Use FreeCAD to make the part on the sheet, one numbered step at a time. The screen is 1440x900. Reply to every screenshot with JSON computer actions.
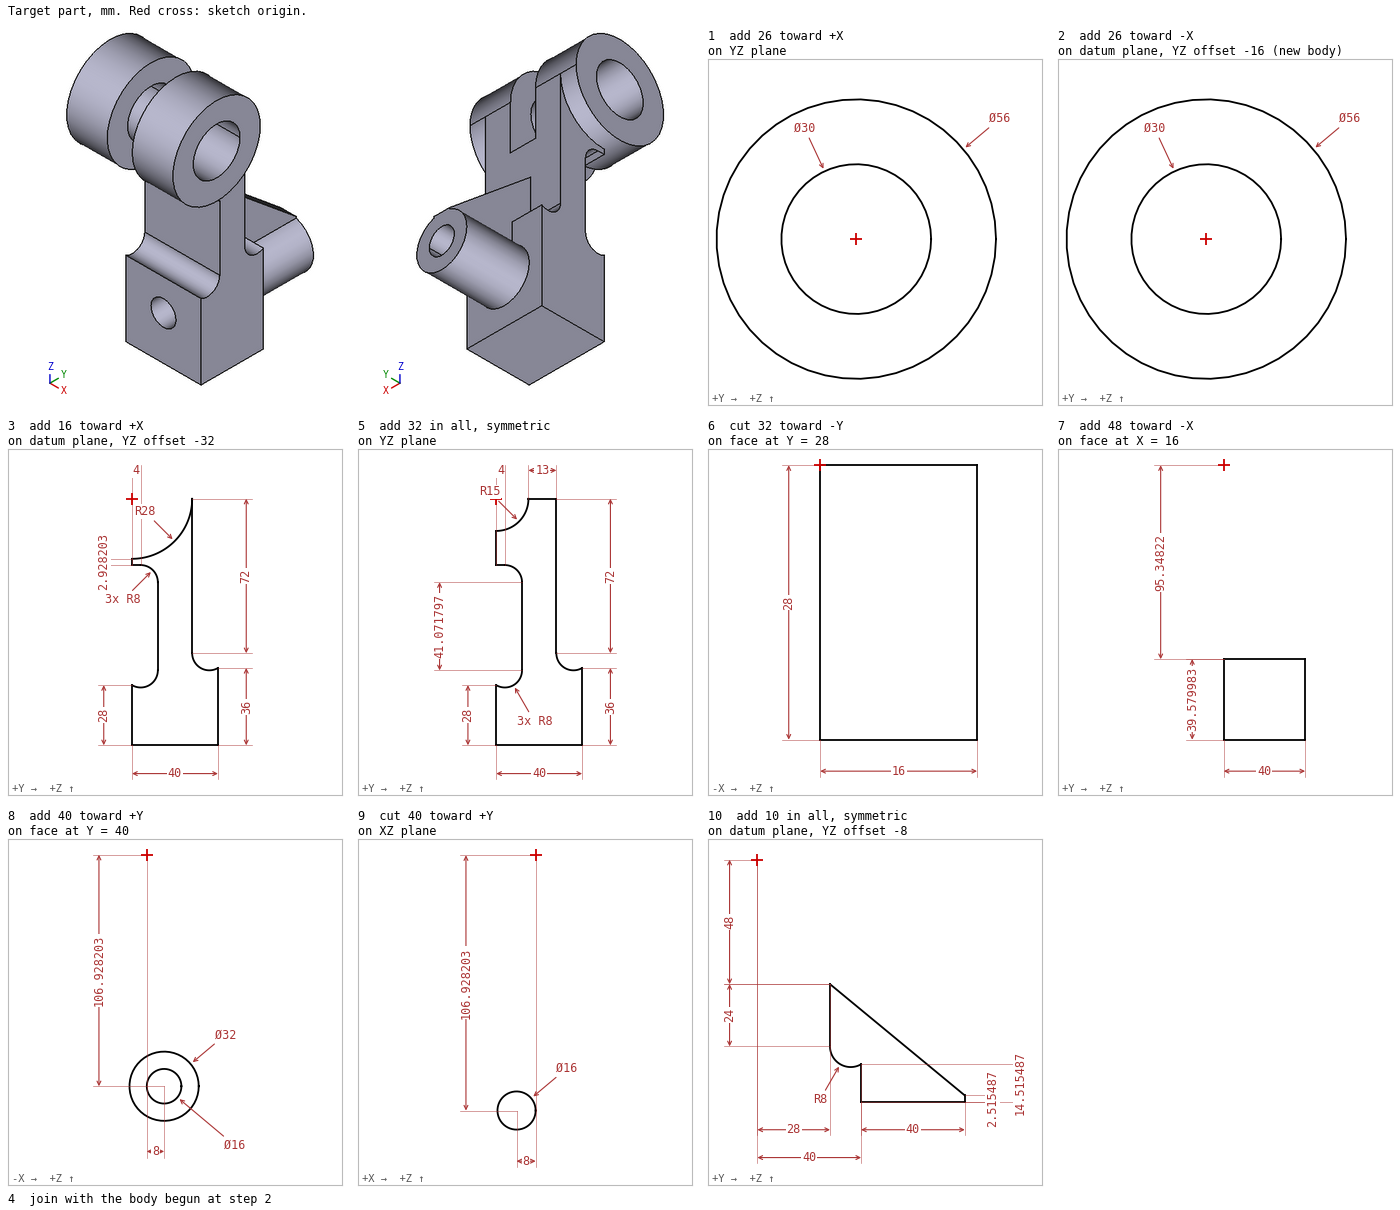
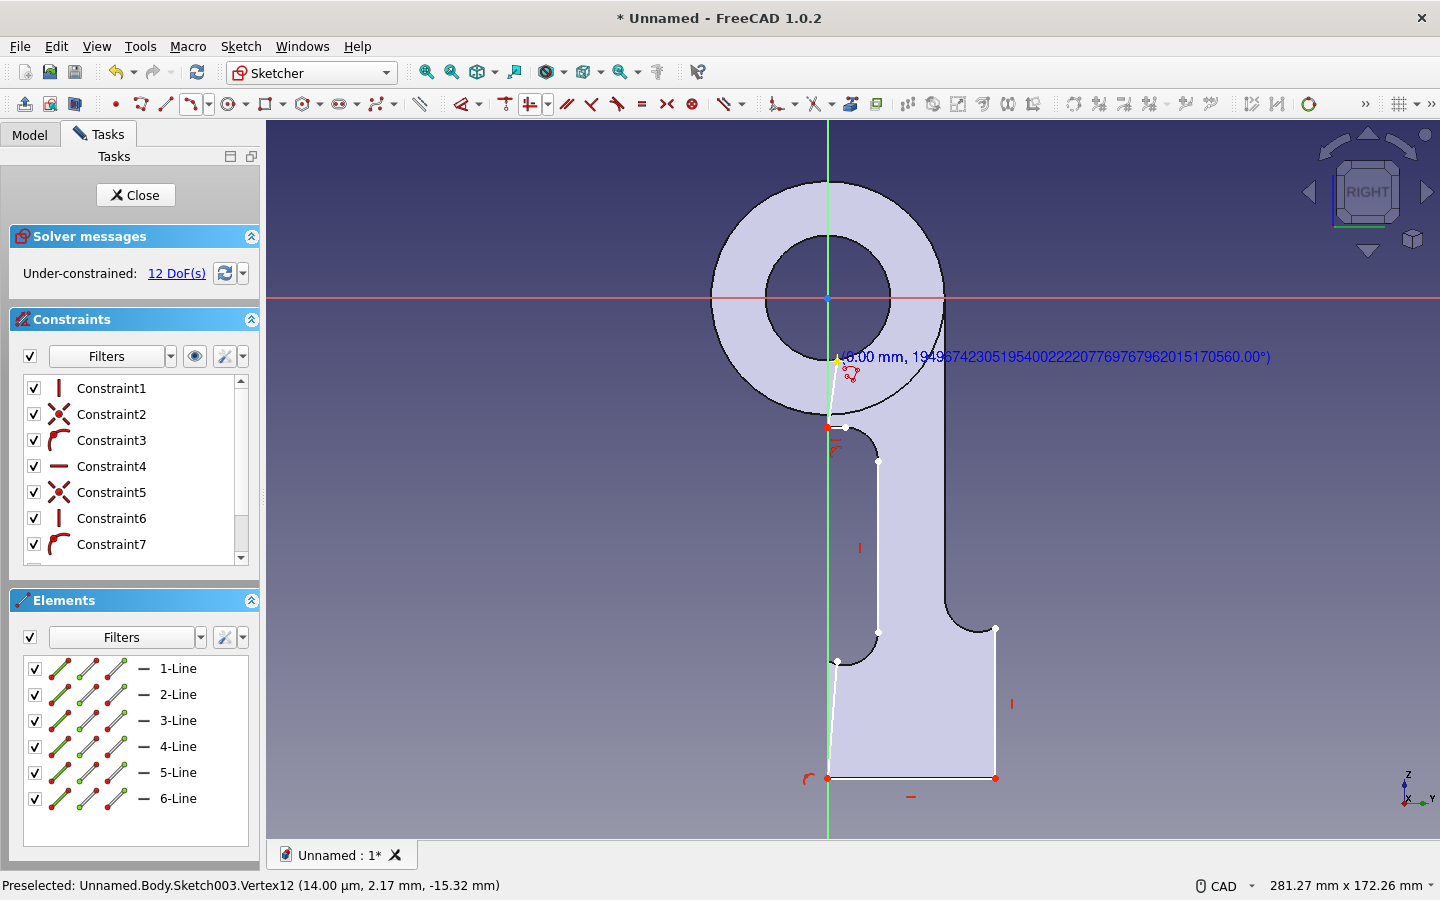
{"action": "left_click", "coordinate": [891, 298]}
{"action": "left_click", "coordinate": [945, 307]}
{"action": "left_click", "coordinate": [945, 599]}
{"action": "right_click", "coordinate": [945, 599]}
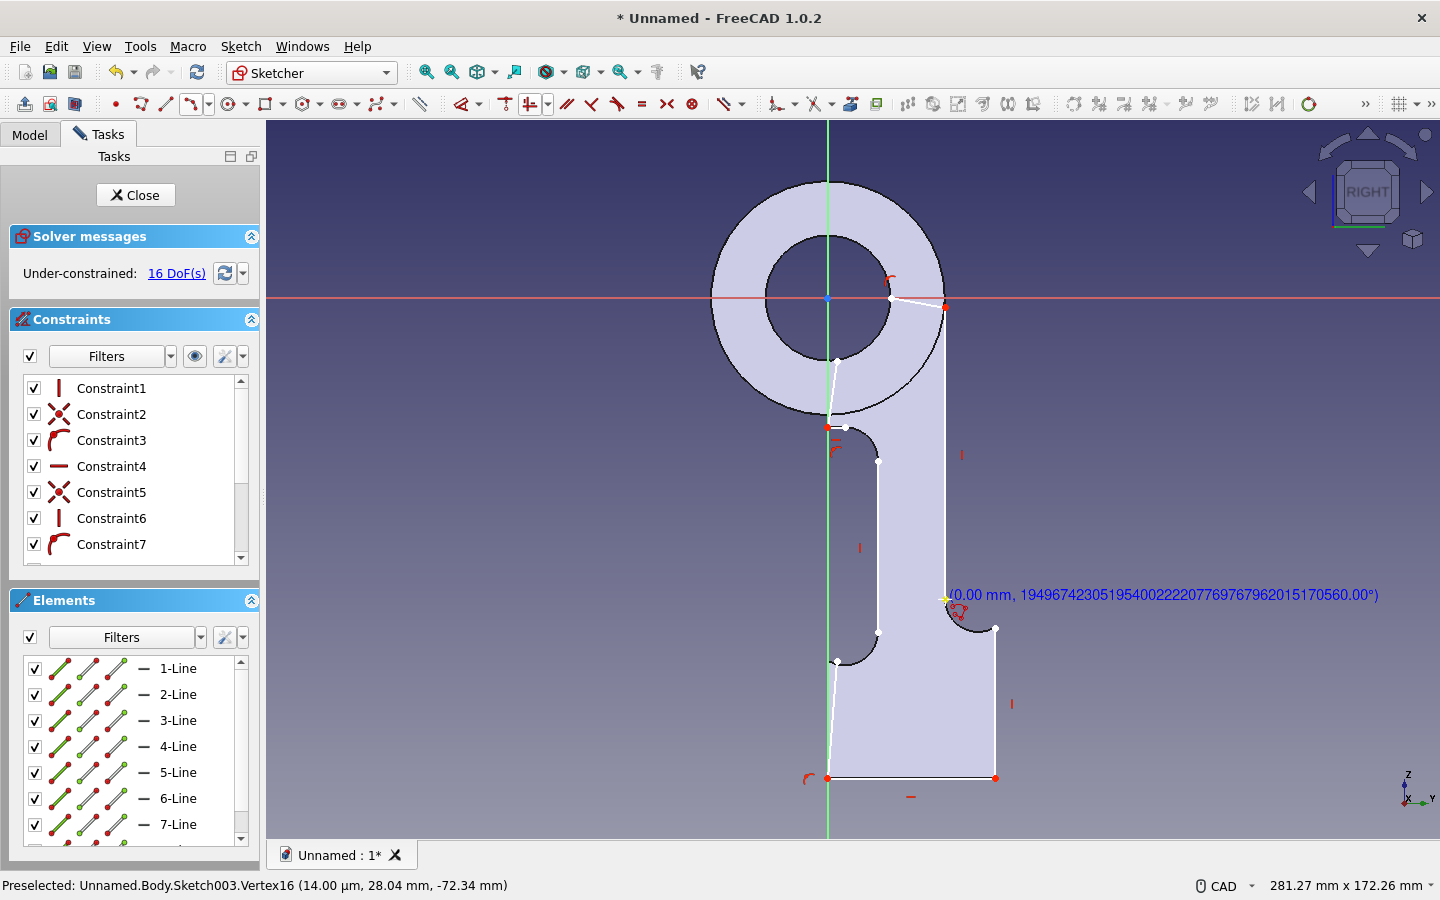
{"action": "left_click", "coordinate": [190, 104]}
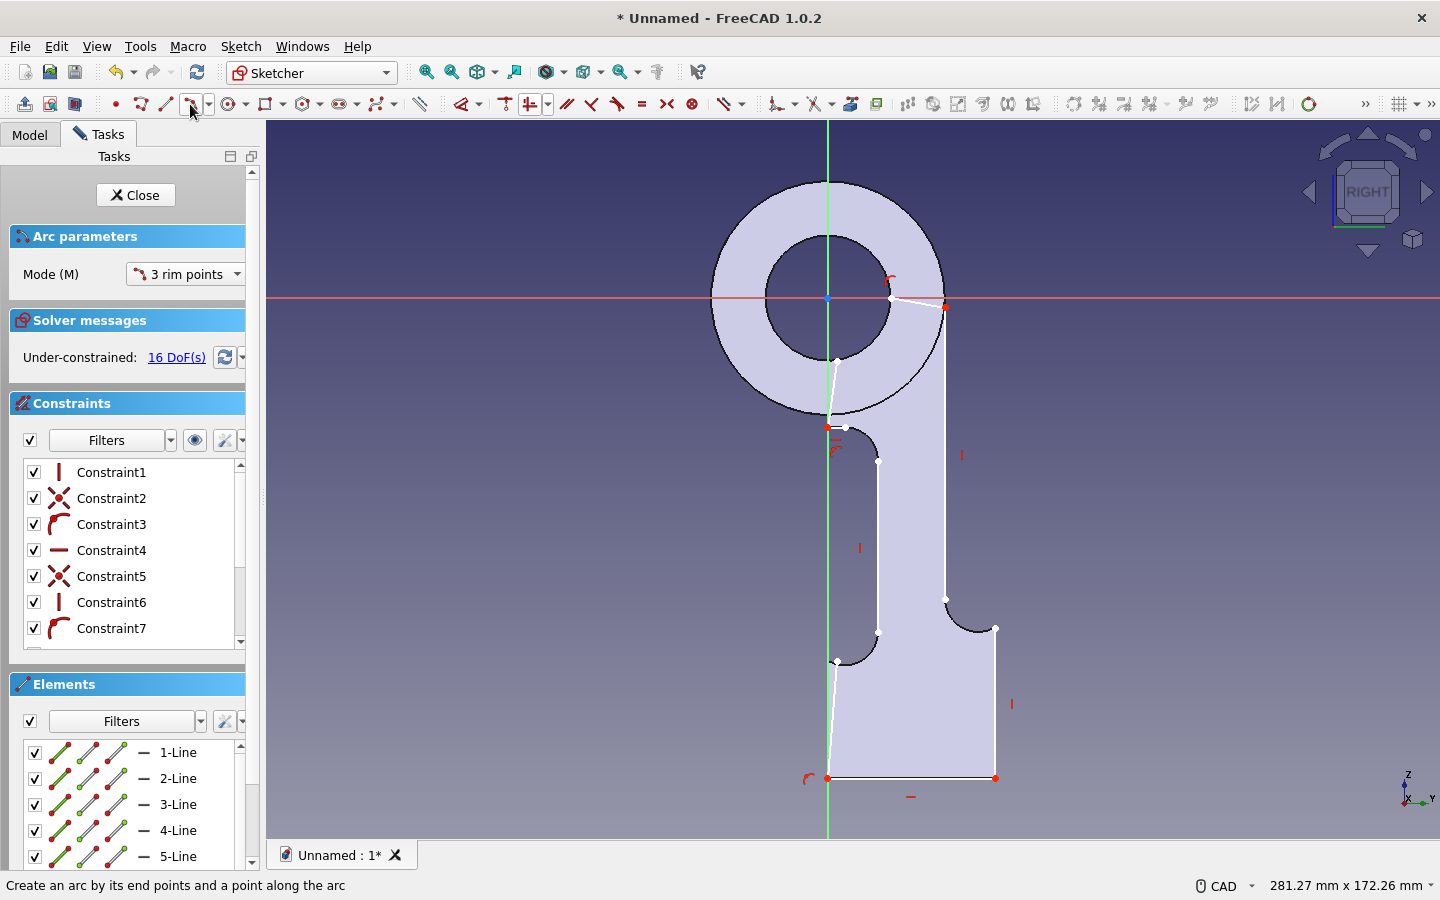
{"action": "left_click", "coordinate": [837, 662]}
{"action": "left_click", "coordinate": [878, 633]}
{"action": "left_click", "coordinate": [861, 661]}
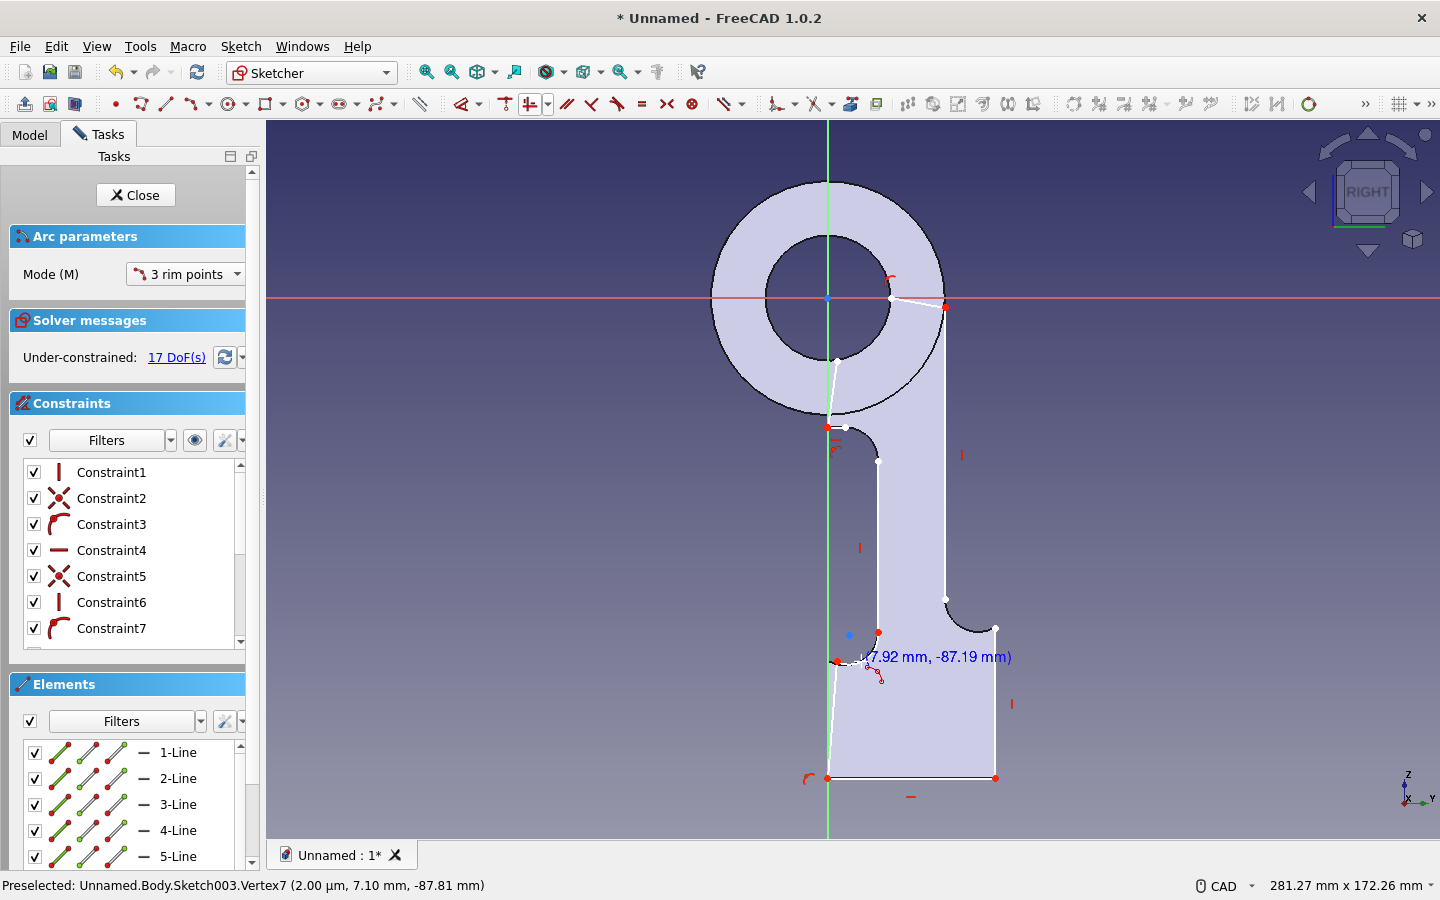
{"action": "left_click", "coordinate": [878, 462]}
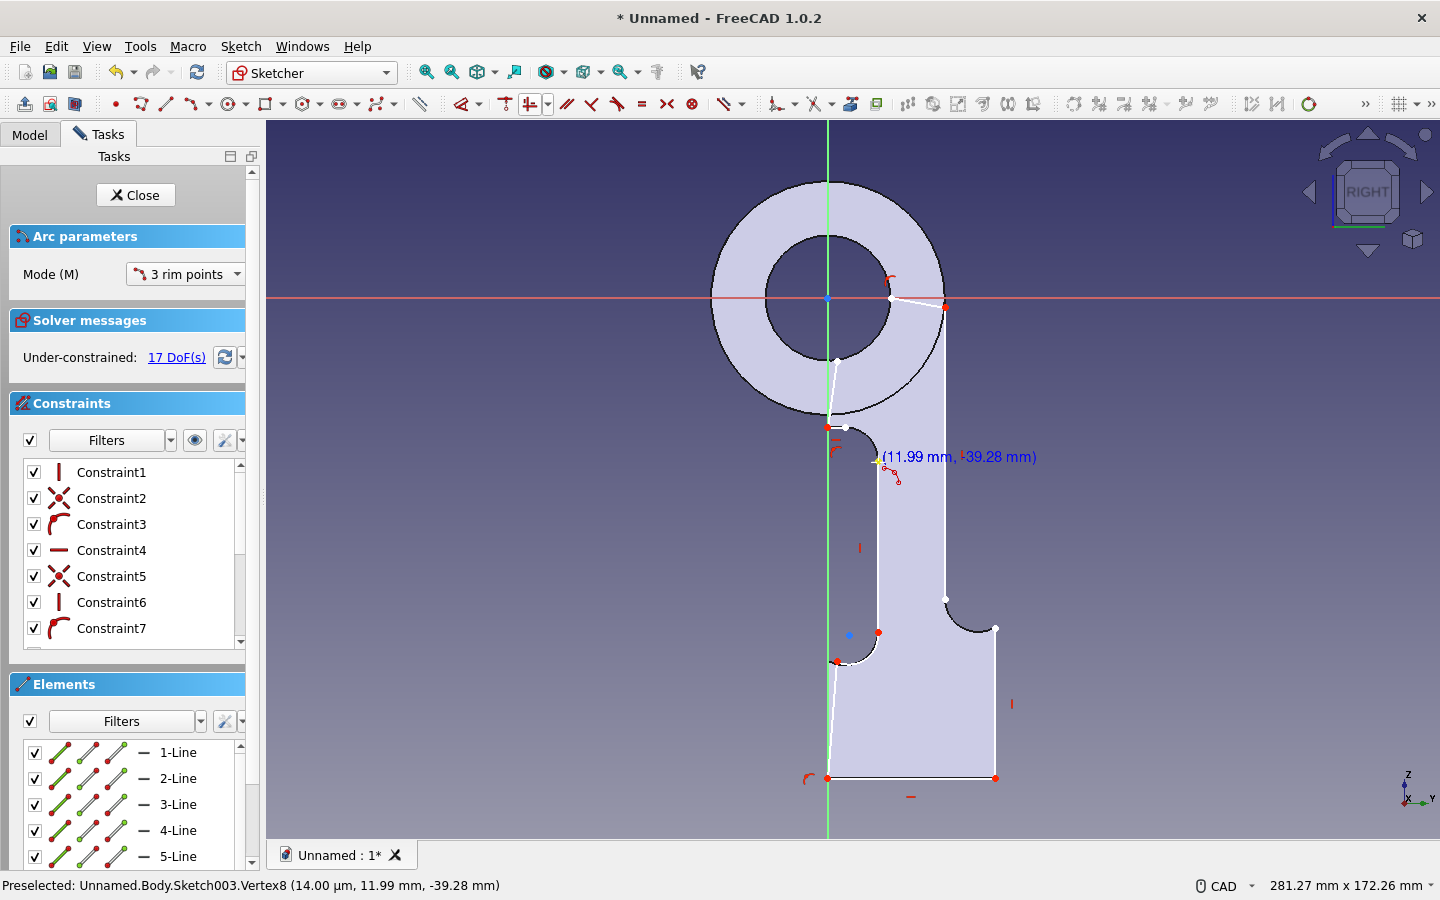
{"action": "scroll", "coordinate": [845, 427], "scroll_direction": "up", "scroll_amount": 4}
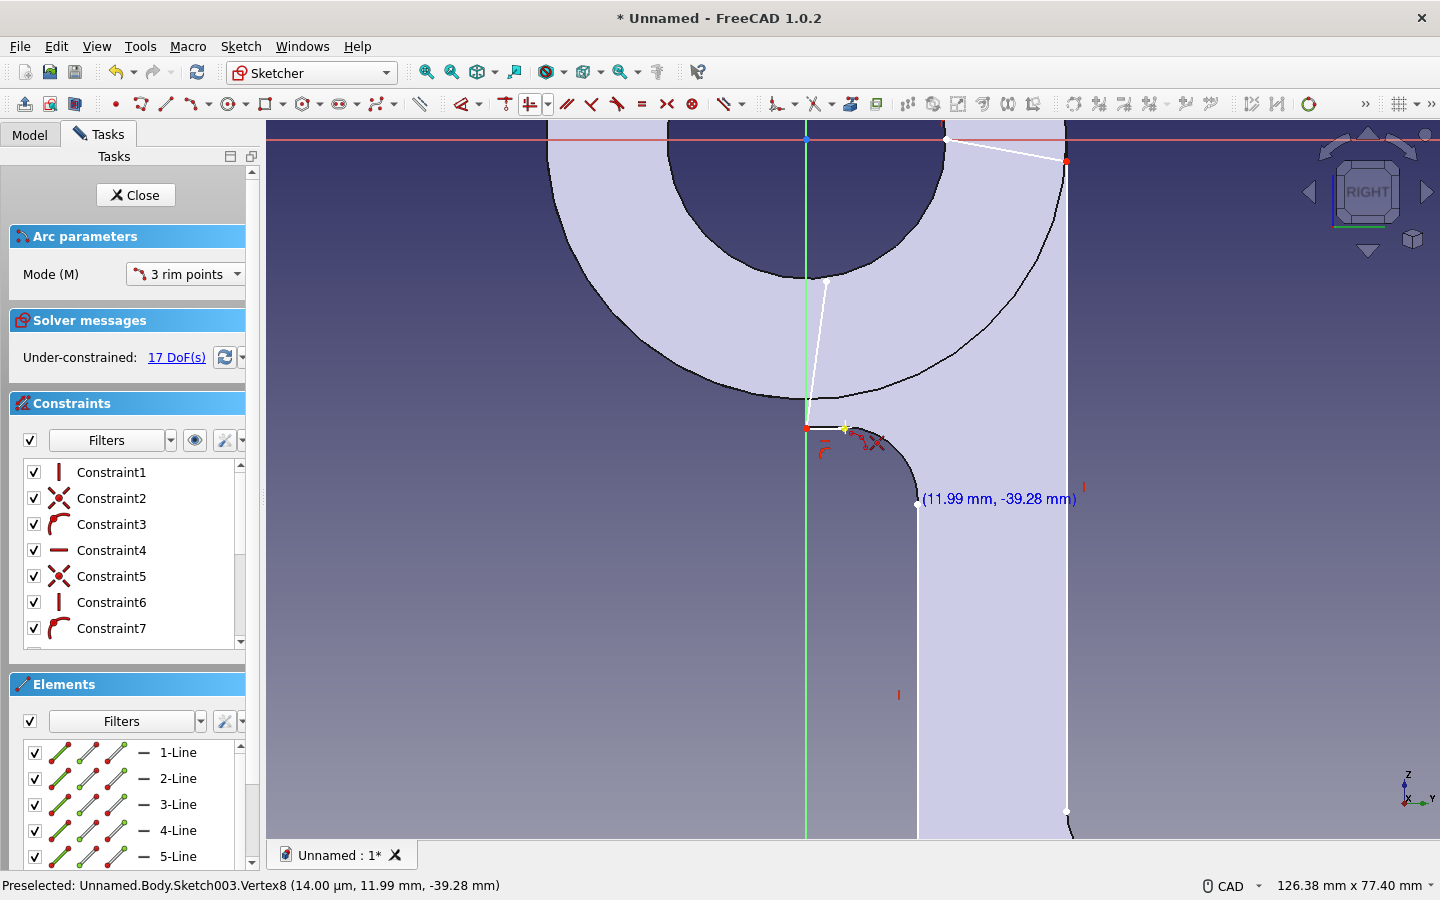
{"action": "left_click", "coordinate": [844, 429]}
{"action": "left_click", "coordinate": [896, 449]}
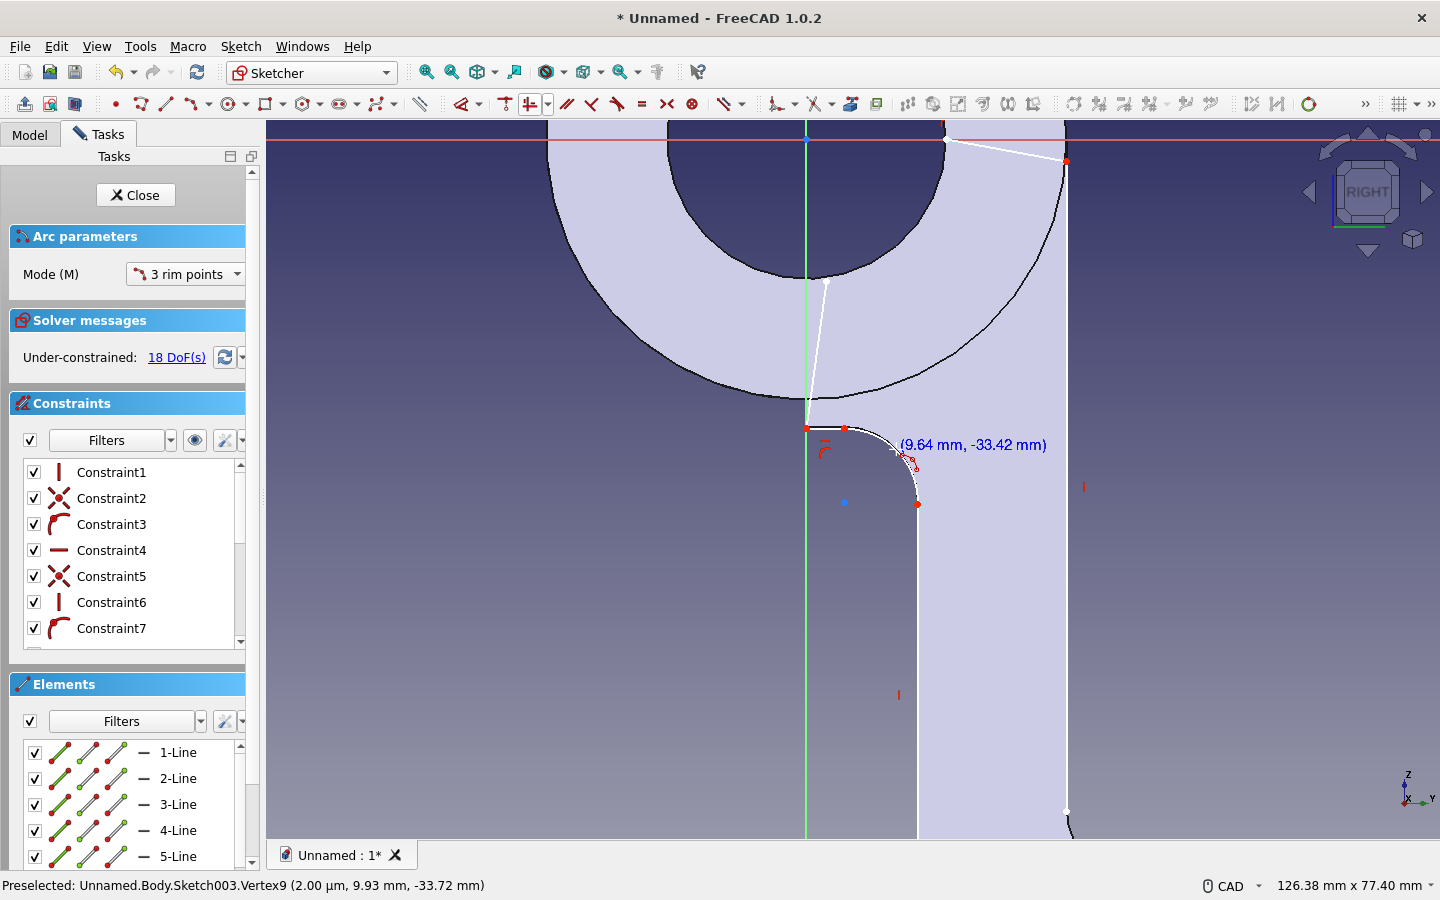
{"action": "left_click", "coordinate": [827, 282]}